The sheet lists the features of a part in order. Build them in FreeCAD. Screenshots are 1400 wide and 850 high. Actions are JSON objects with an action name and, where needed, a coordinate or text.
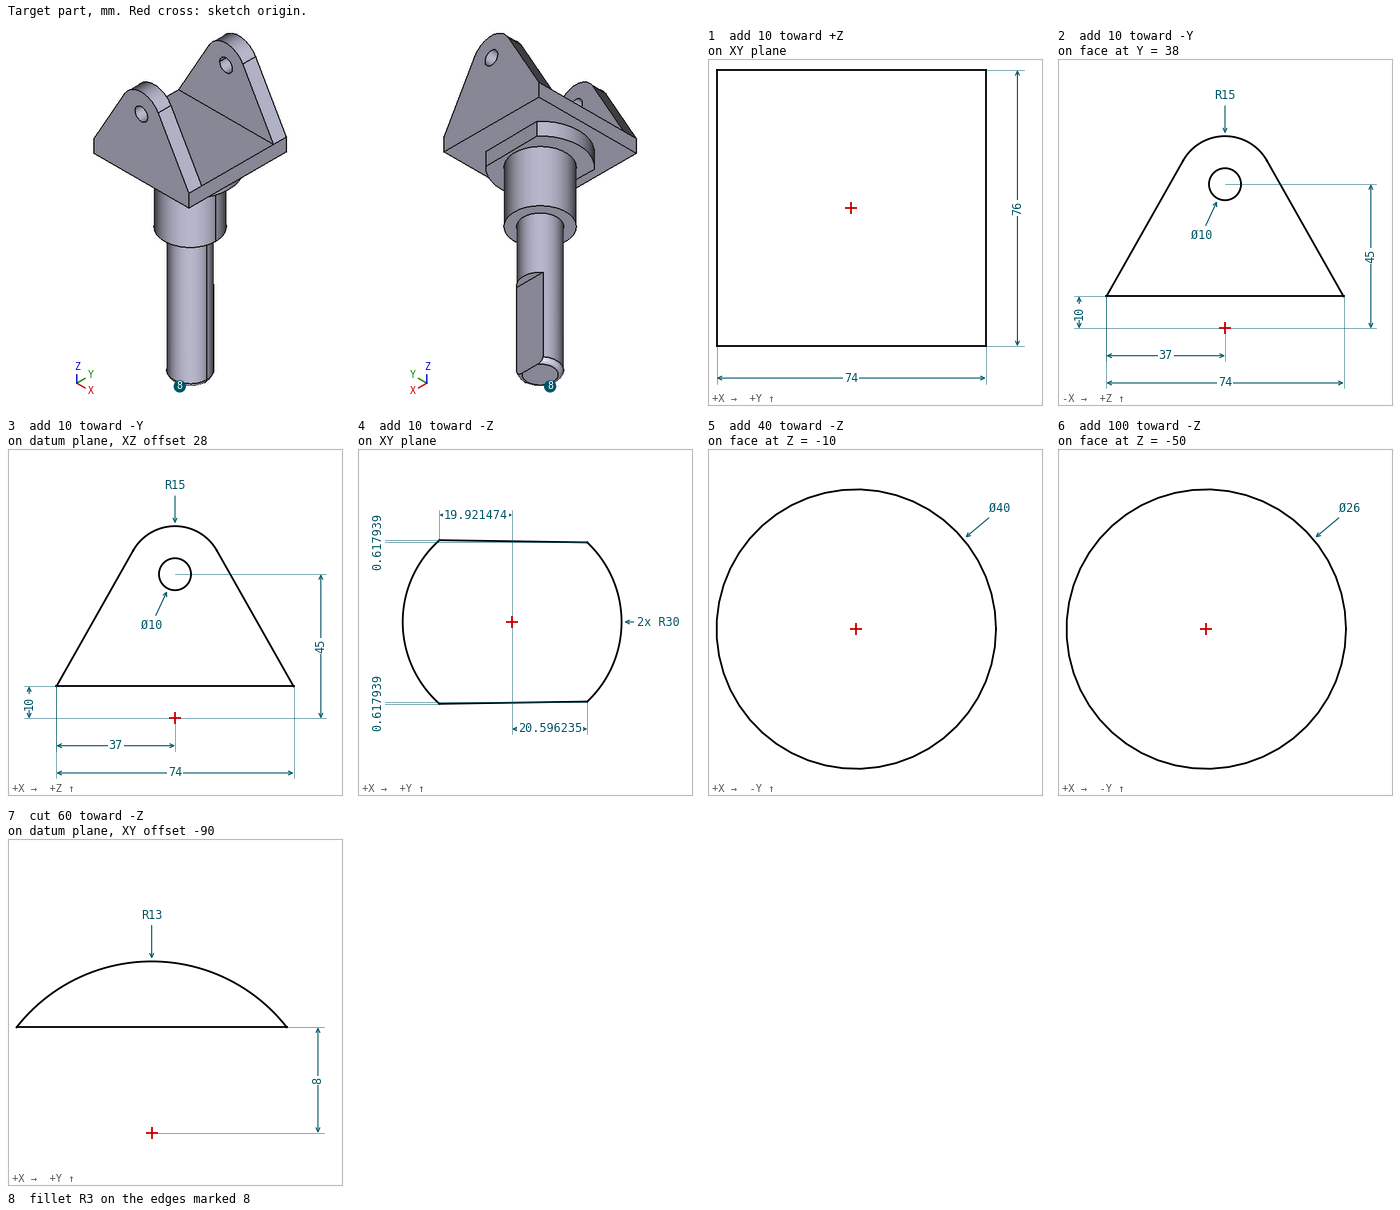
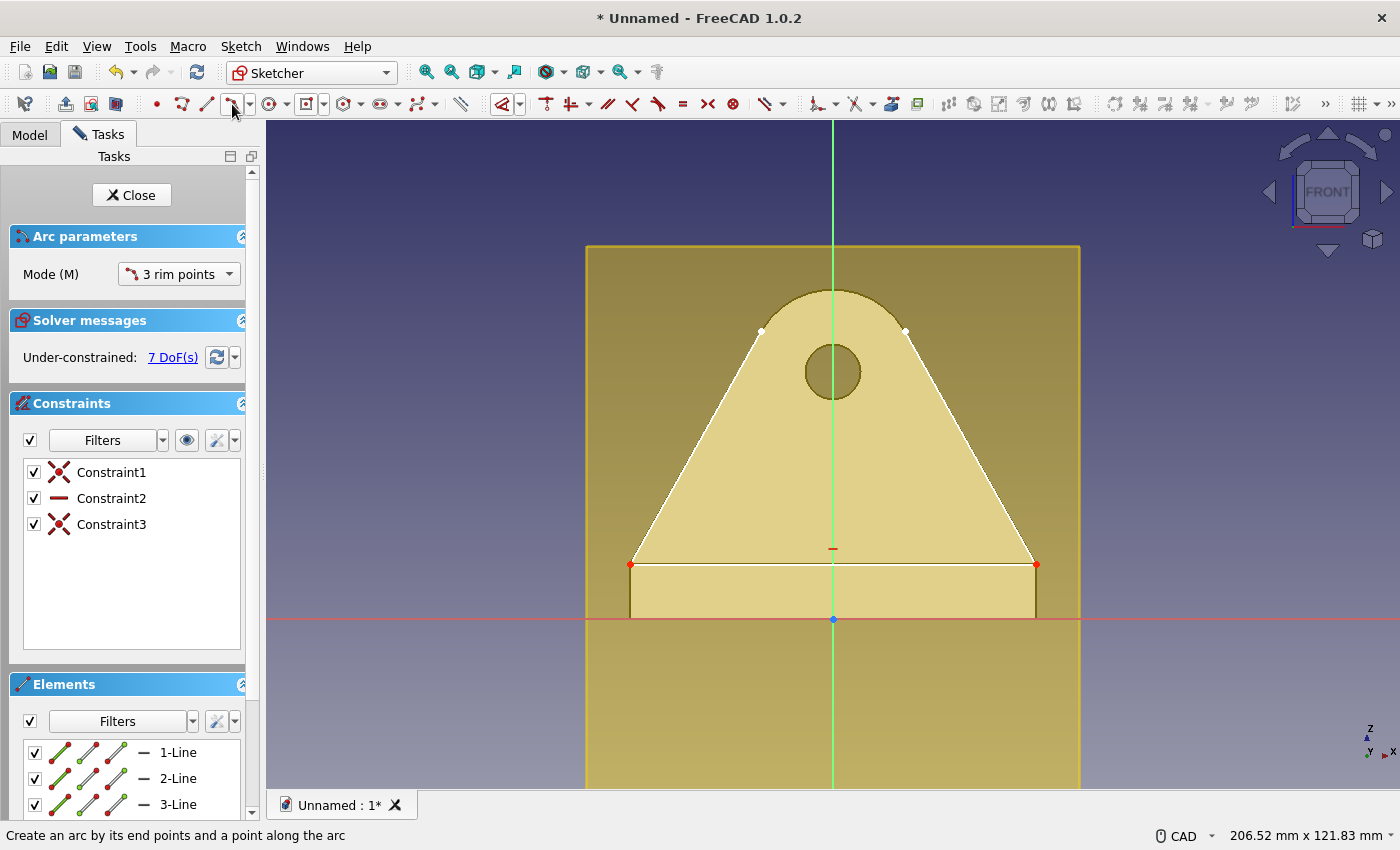
{"action": "left_click", "coordinate": [905, 332]}
{"action": "left_click", "coordinate": [761, 332]}
{"action": "left_click", "coordinate": [850, 291]}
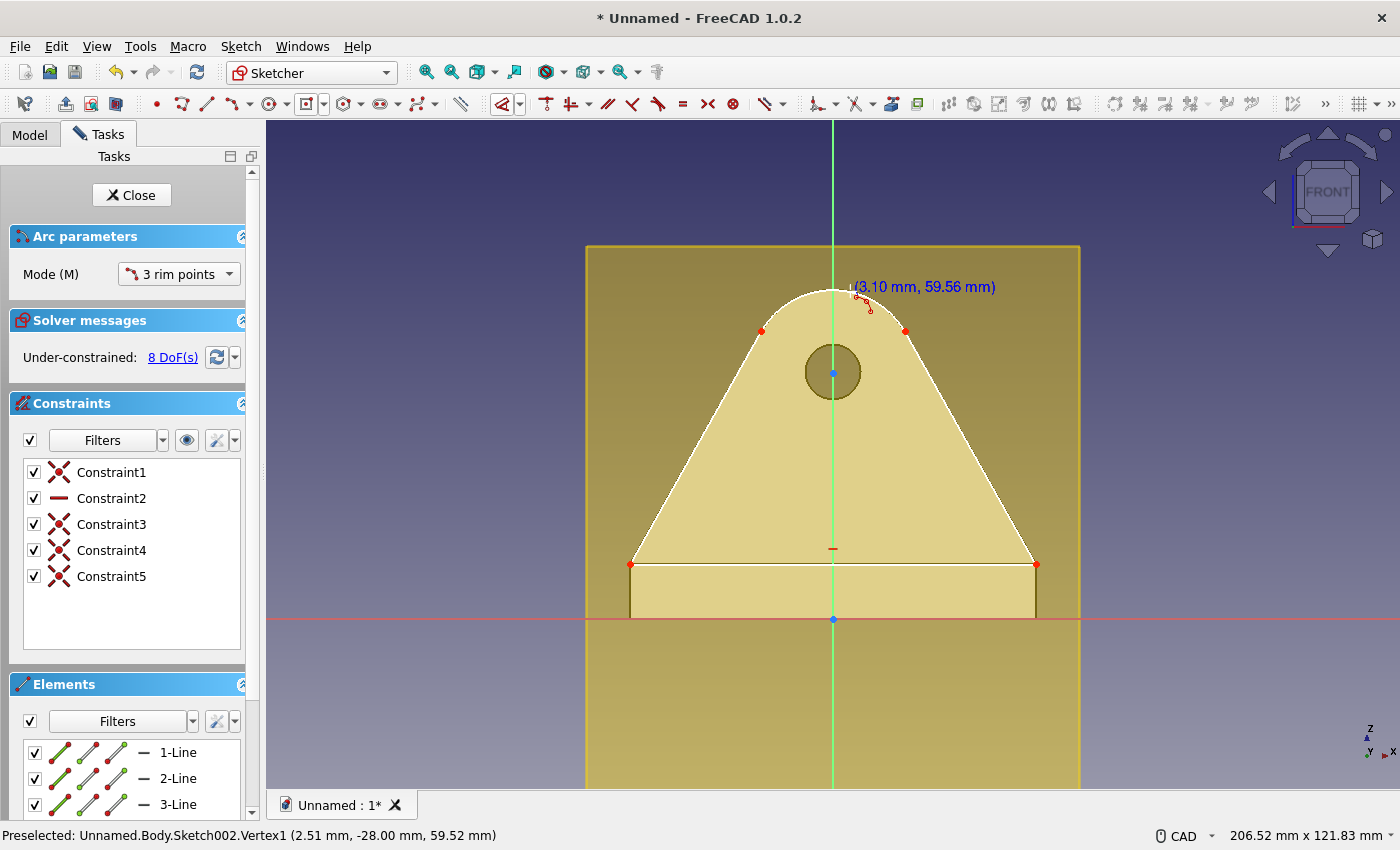
{"action": "key", "text": "g c"}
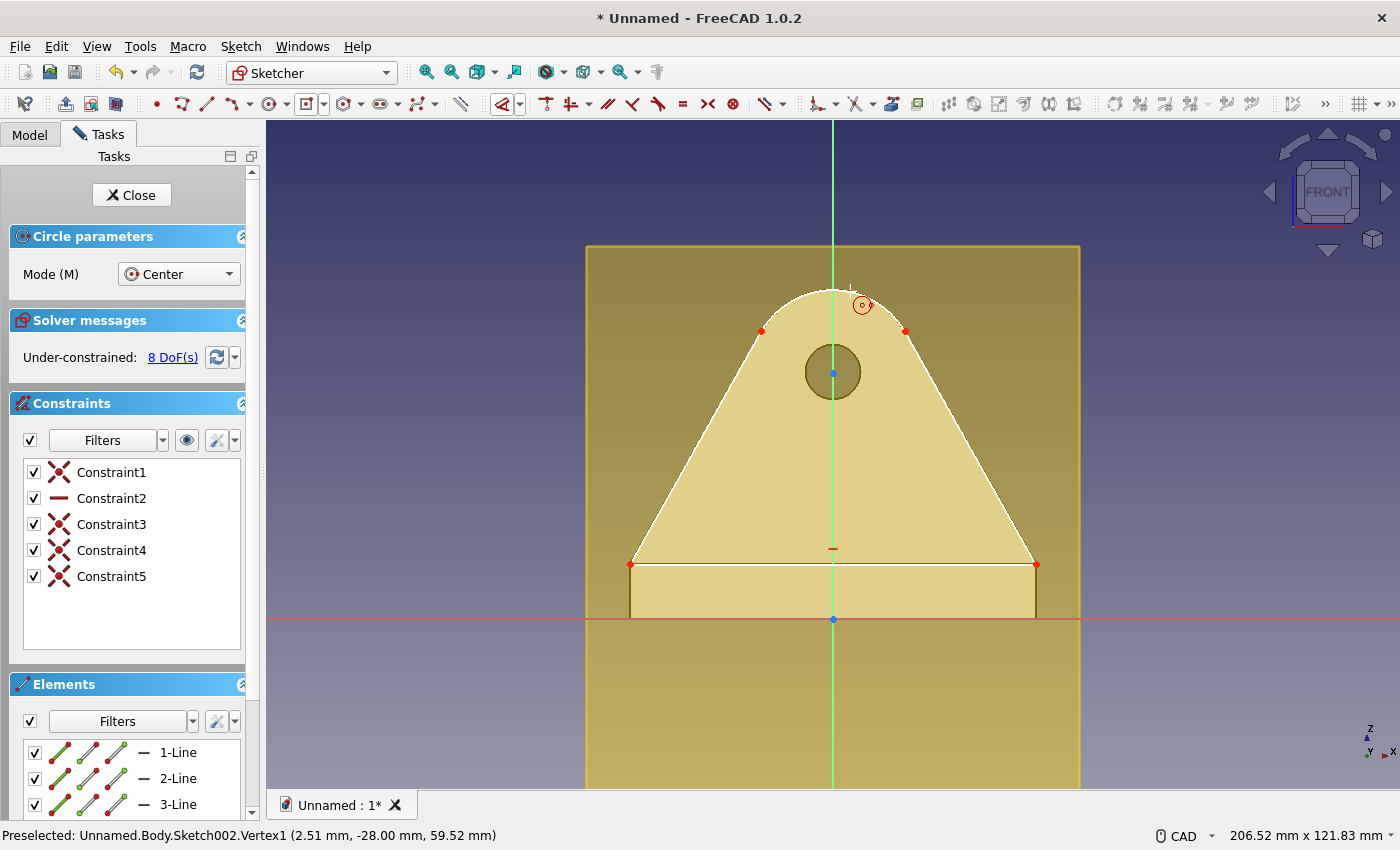
{"action": "left_click", "coordinate": [833, 372]}
{"action": "left_click", "coordinate": [852, 353]}
{"action": "key", "text": "Escape"}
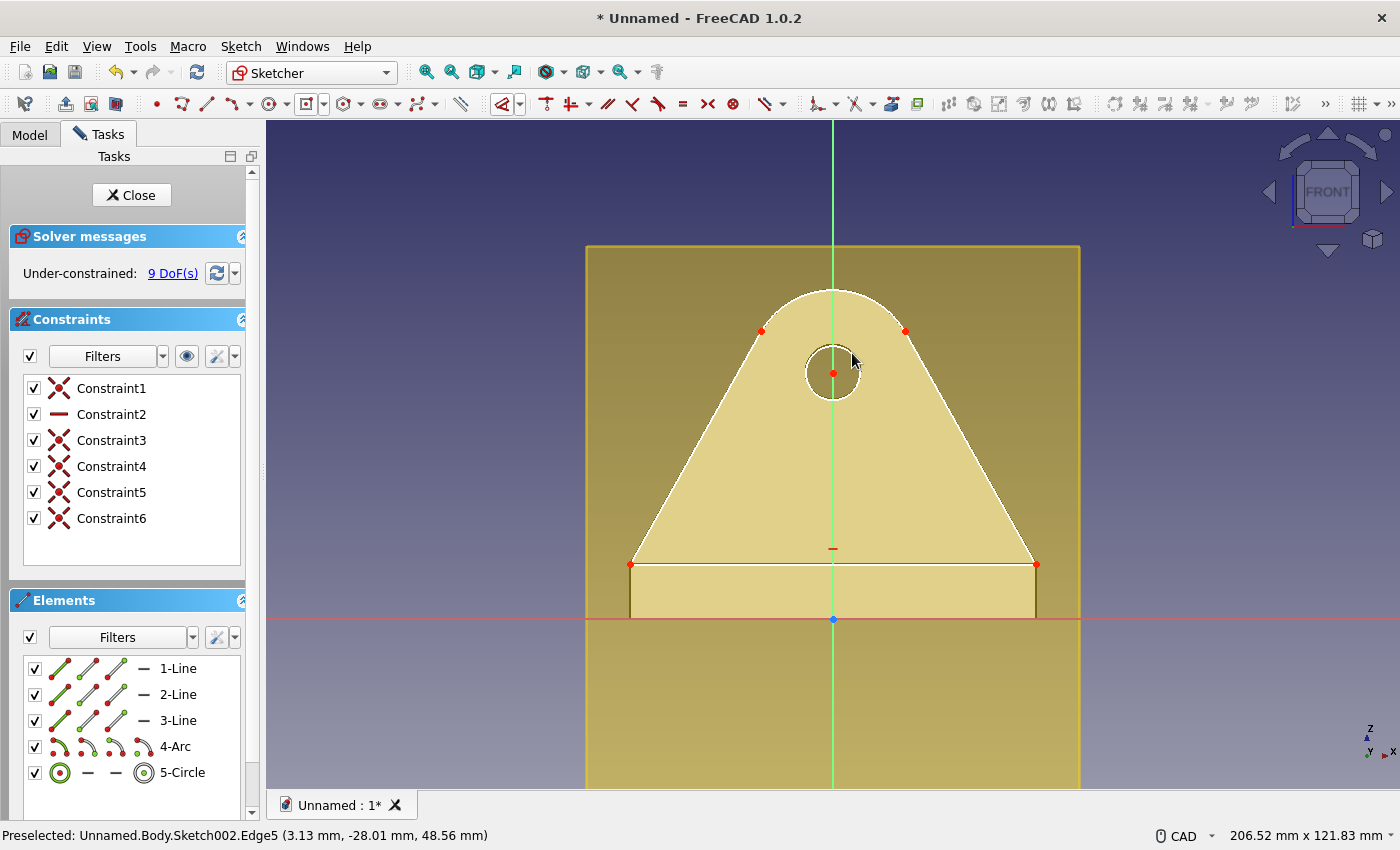
{"action": "left_click", "coordinate": [722, 402]}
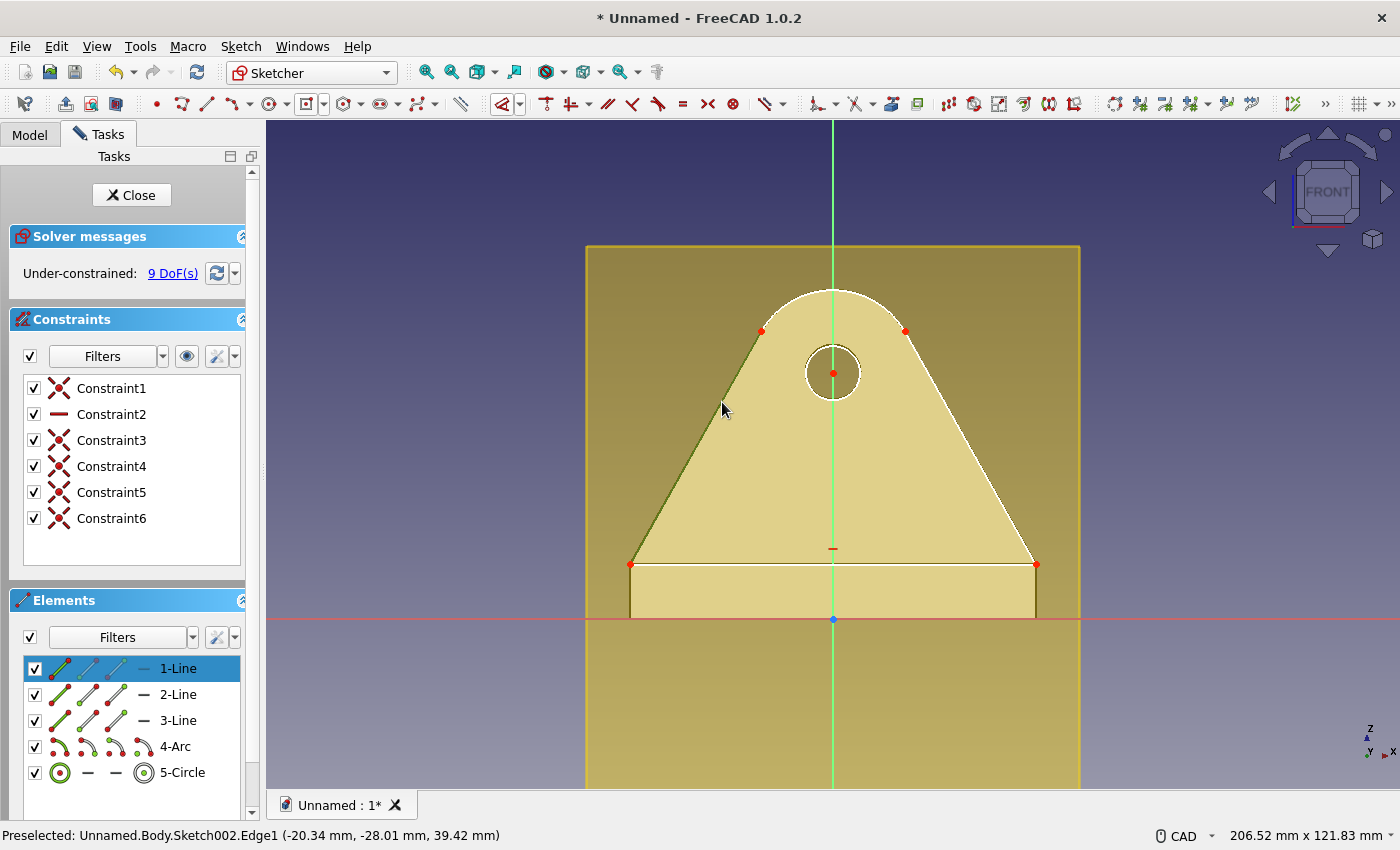
{"action": "left_click", "coordinate": [867, 297]}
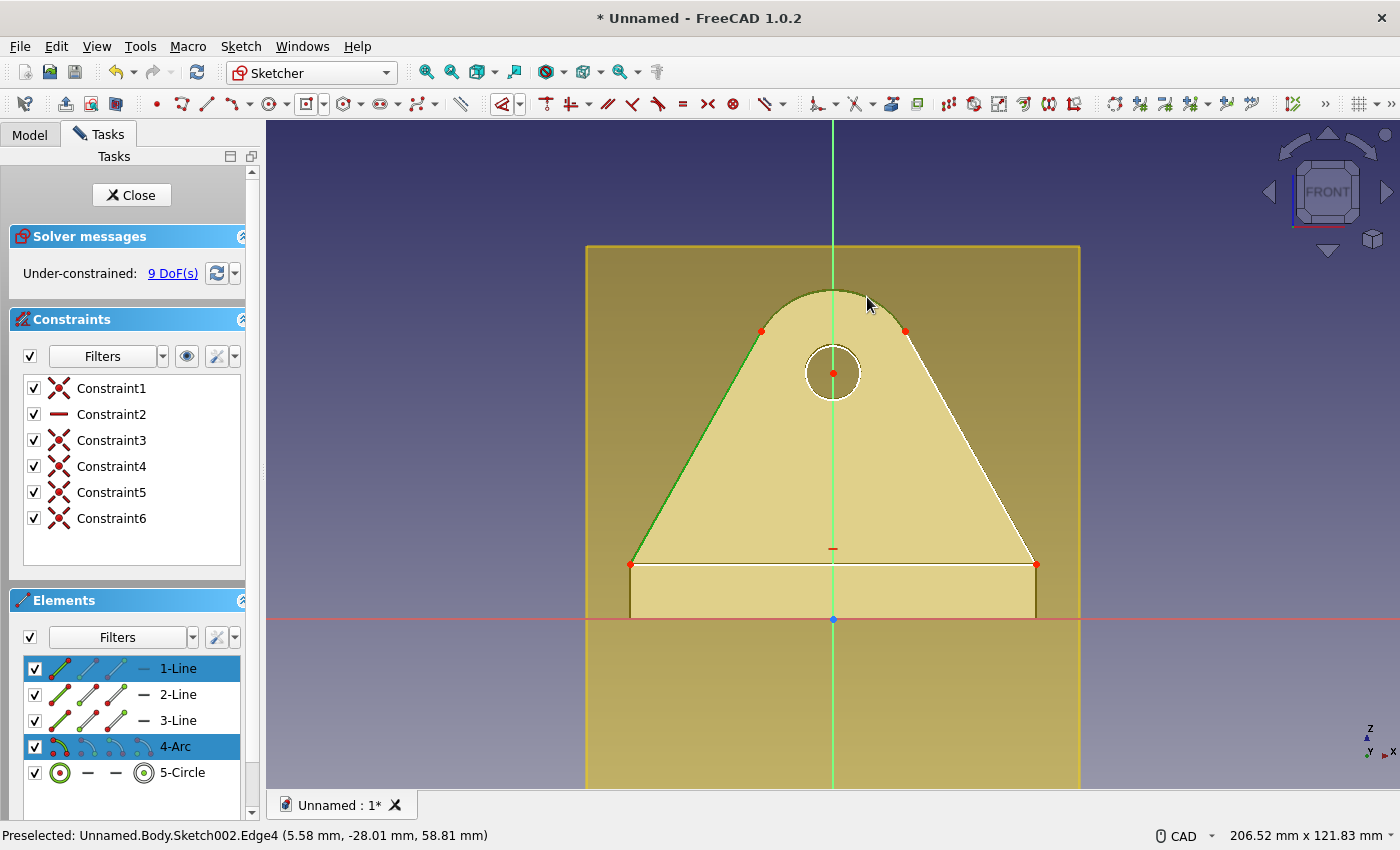
{"action": "left_click", "coordinate": [658, 104]}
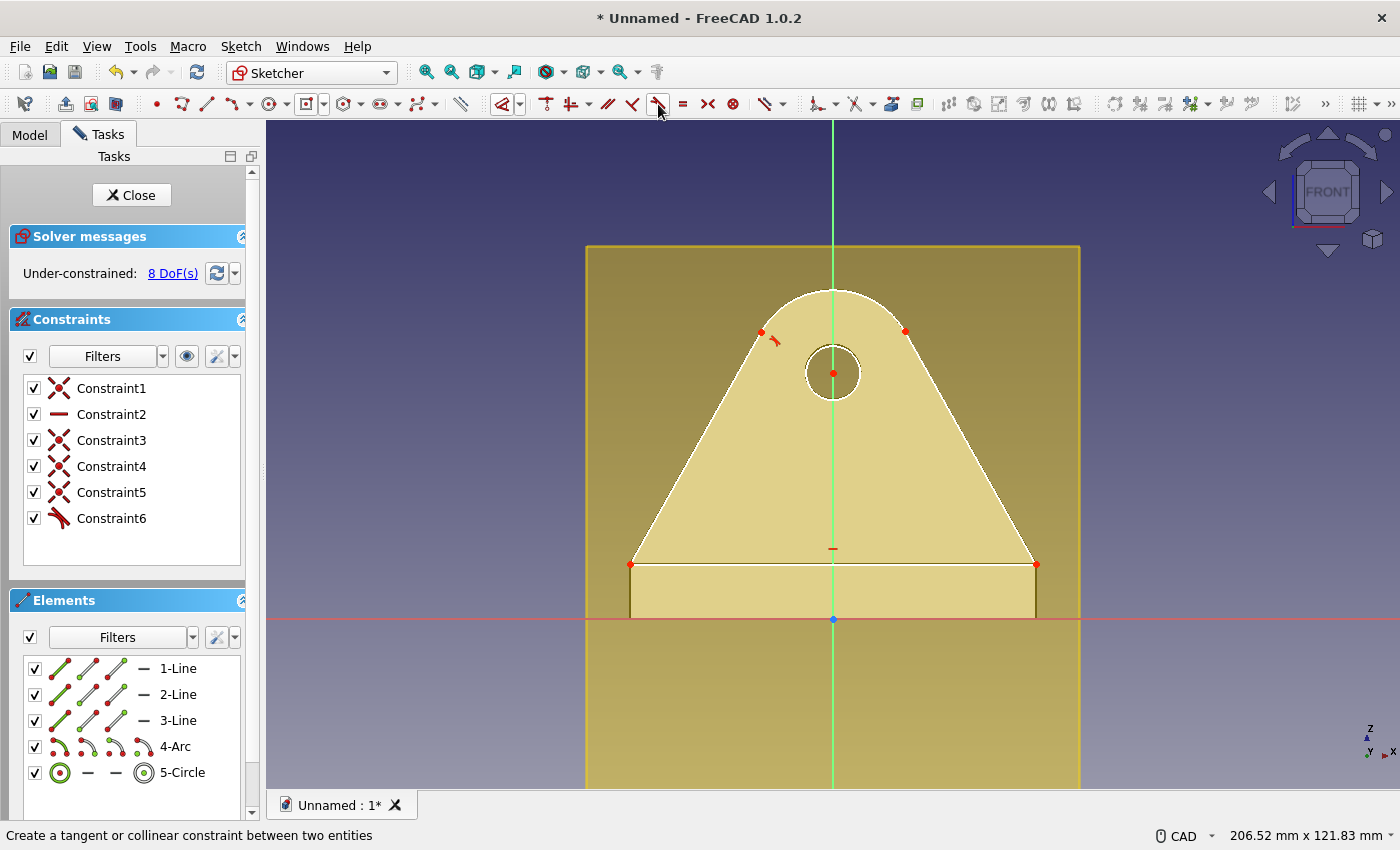
{"action": "left_click", "coordinate": [997, 495]}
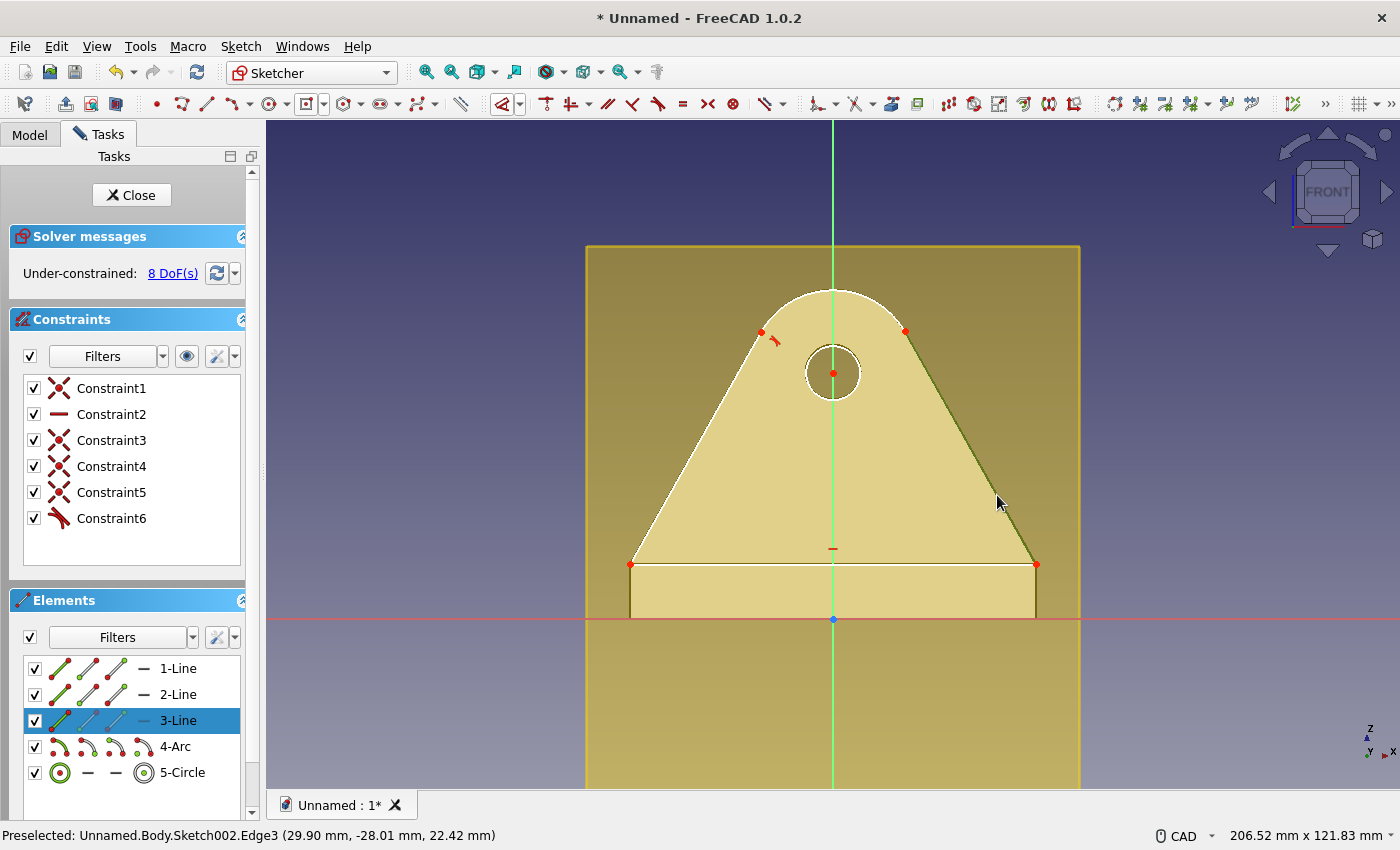
{"action": "left_click", "coordinate": [867, 297]}